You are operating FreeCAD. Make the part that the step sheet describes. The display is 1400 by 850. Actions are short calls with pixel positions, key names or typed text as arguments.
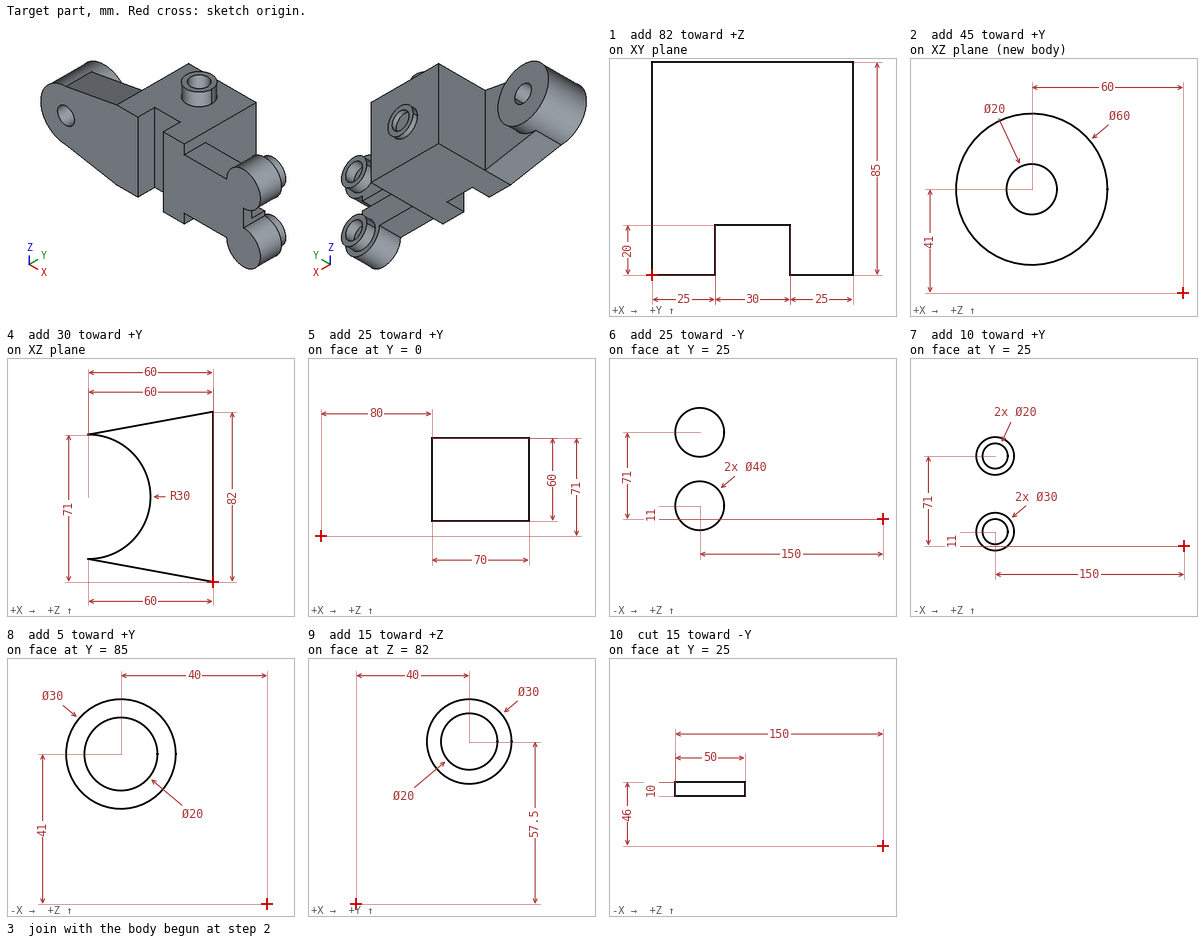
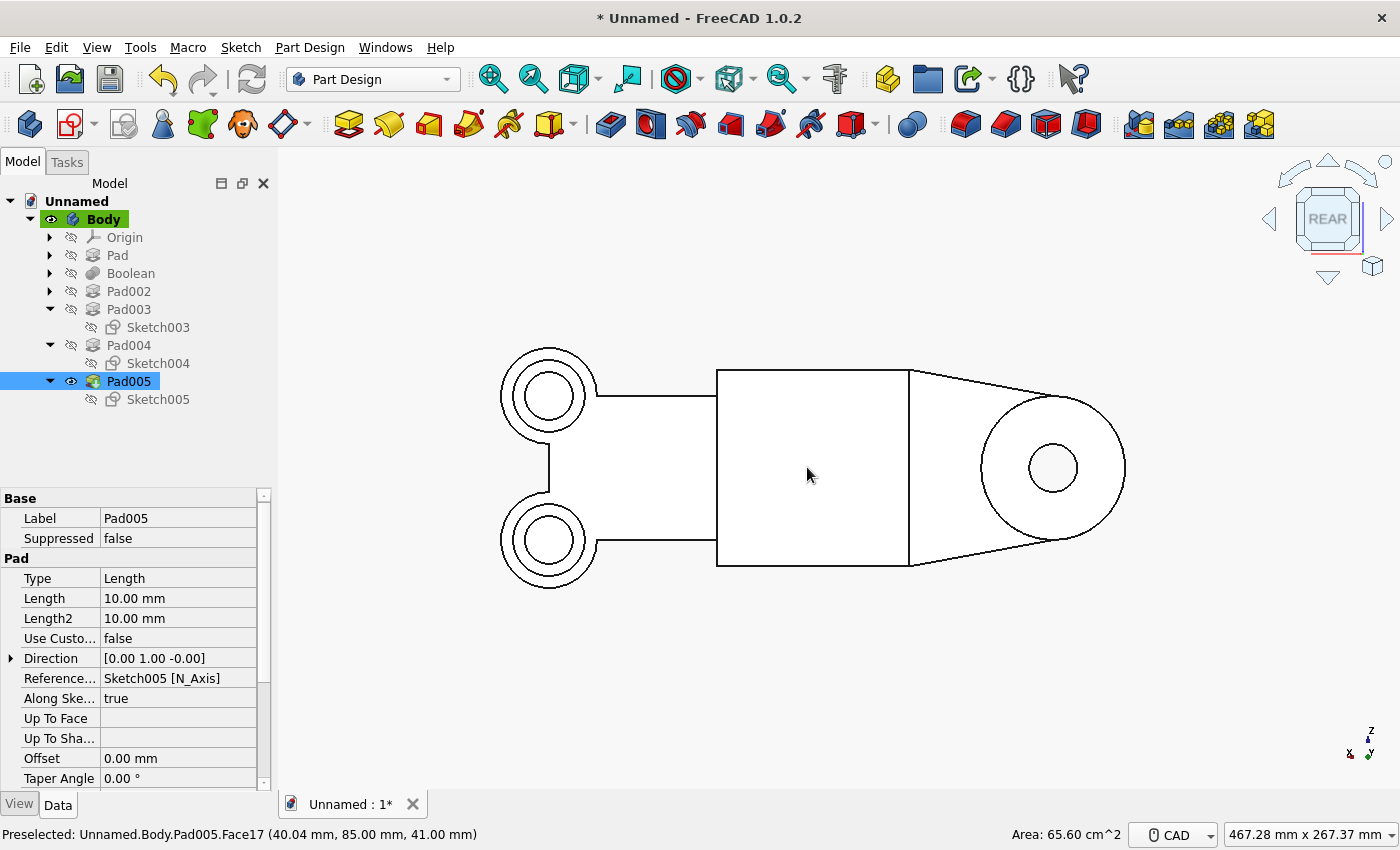
click(70, 124)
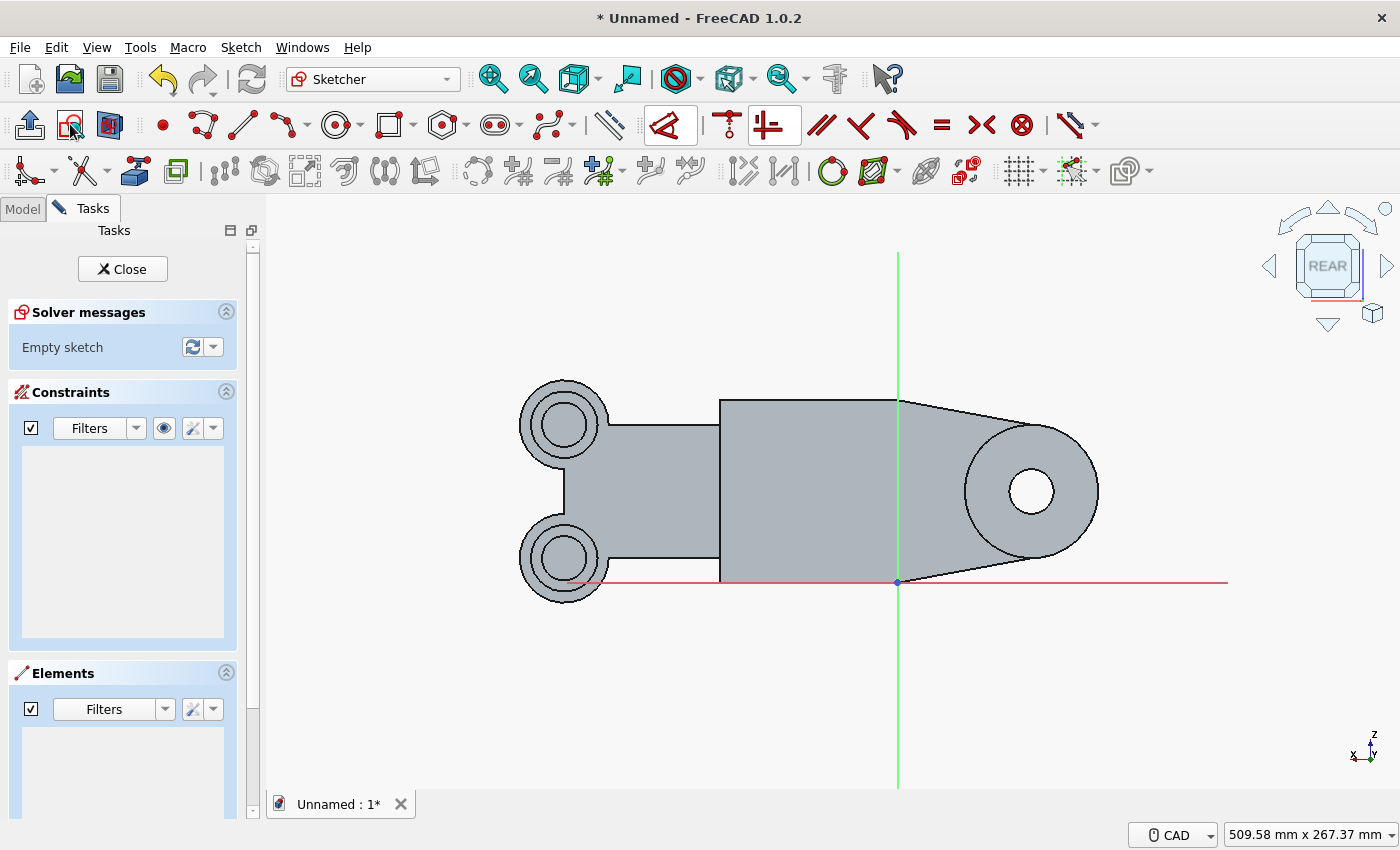
scroll(868, 533, up, 6)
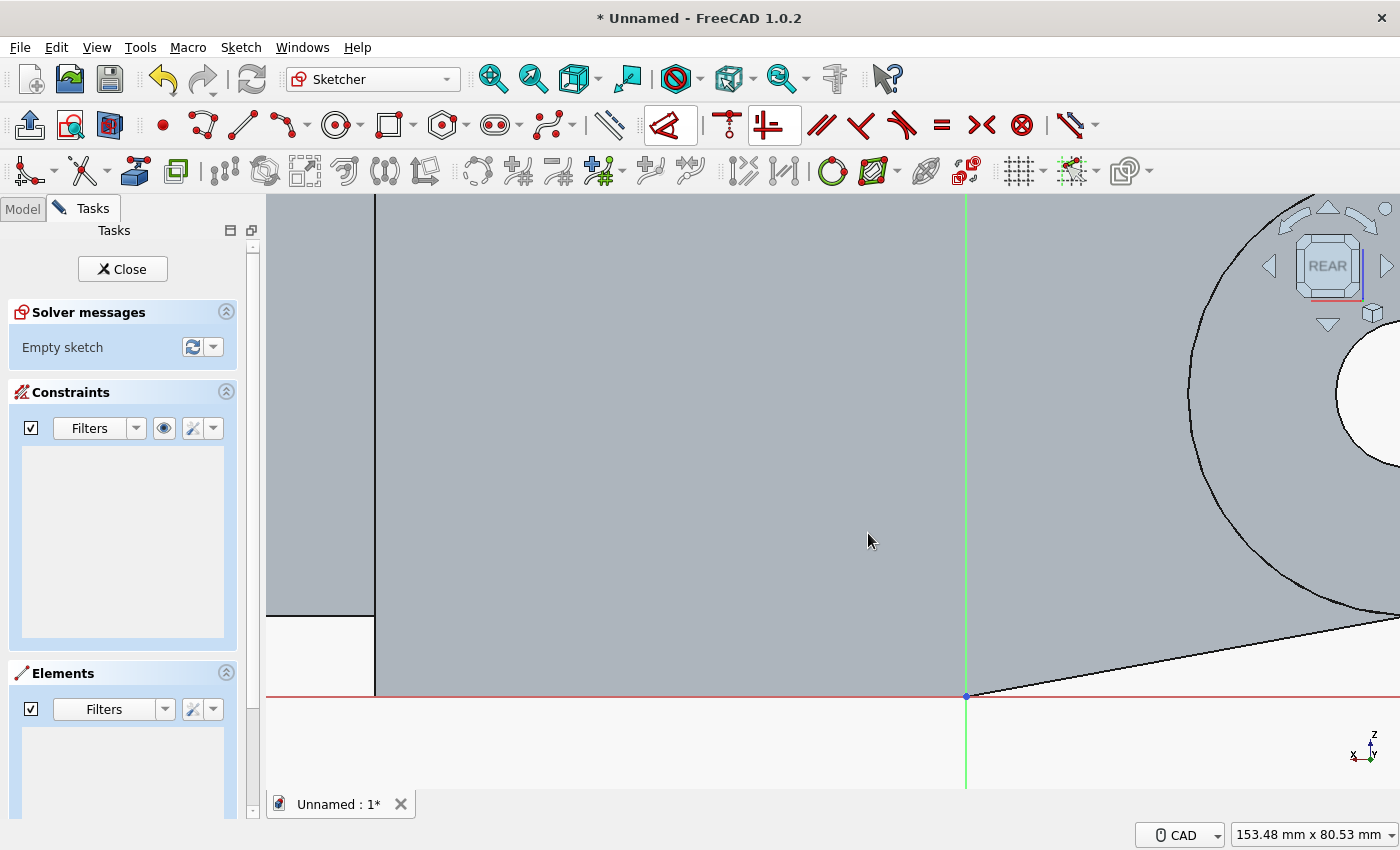
click(336, 126)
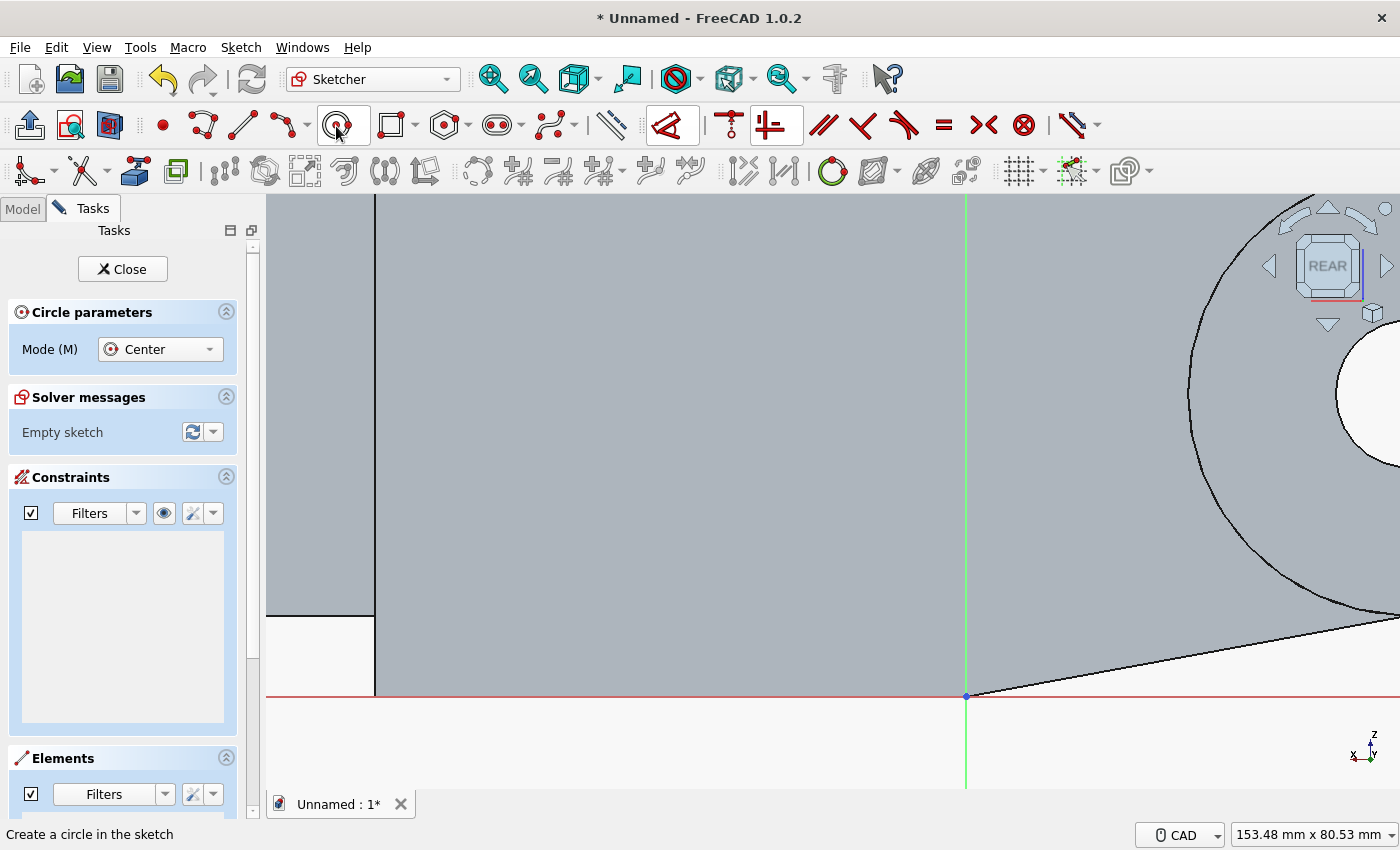
click(671, 394)
click(749, 316)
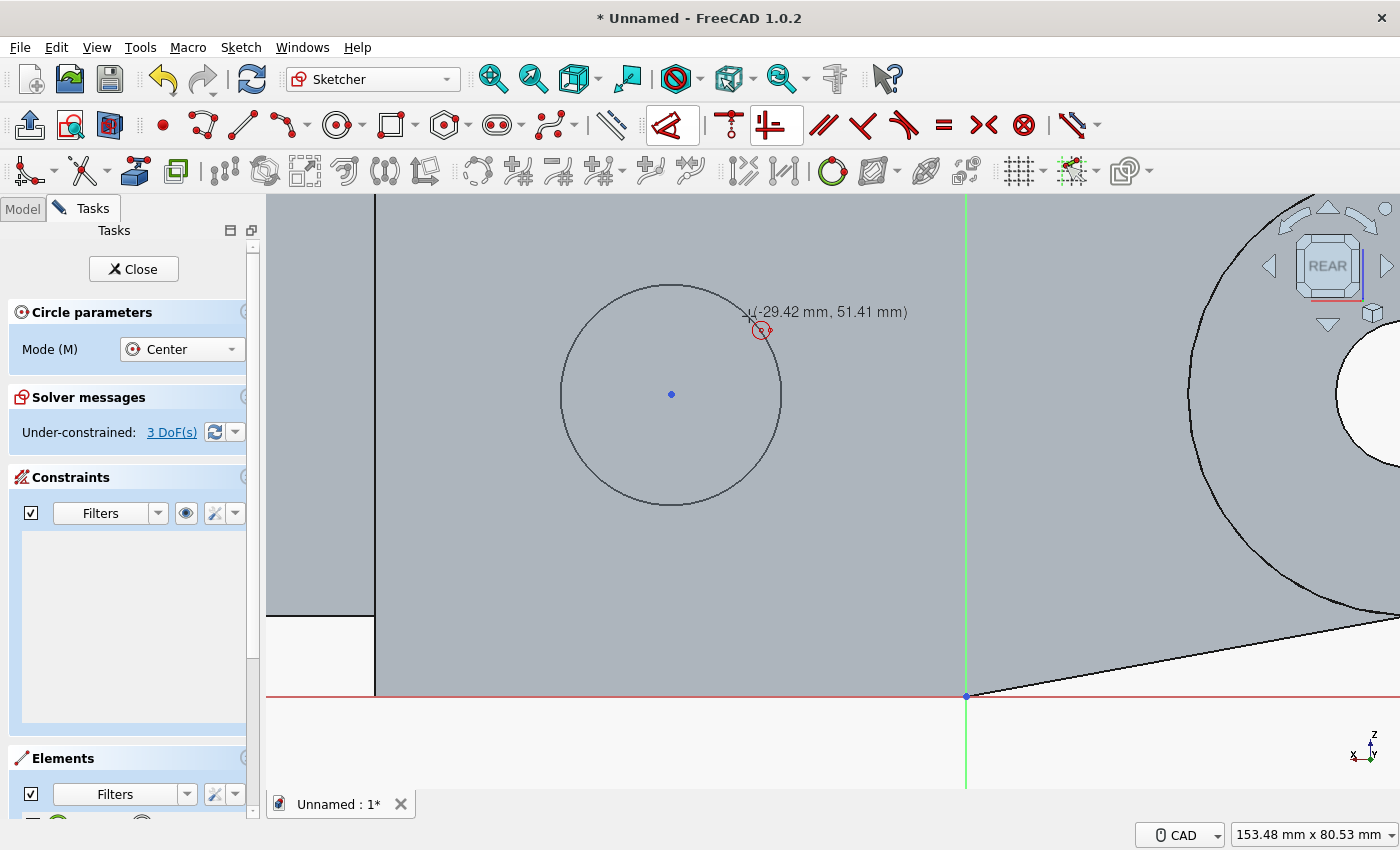
click(671, 395)
click(723, 342)
key(Escape)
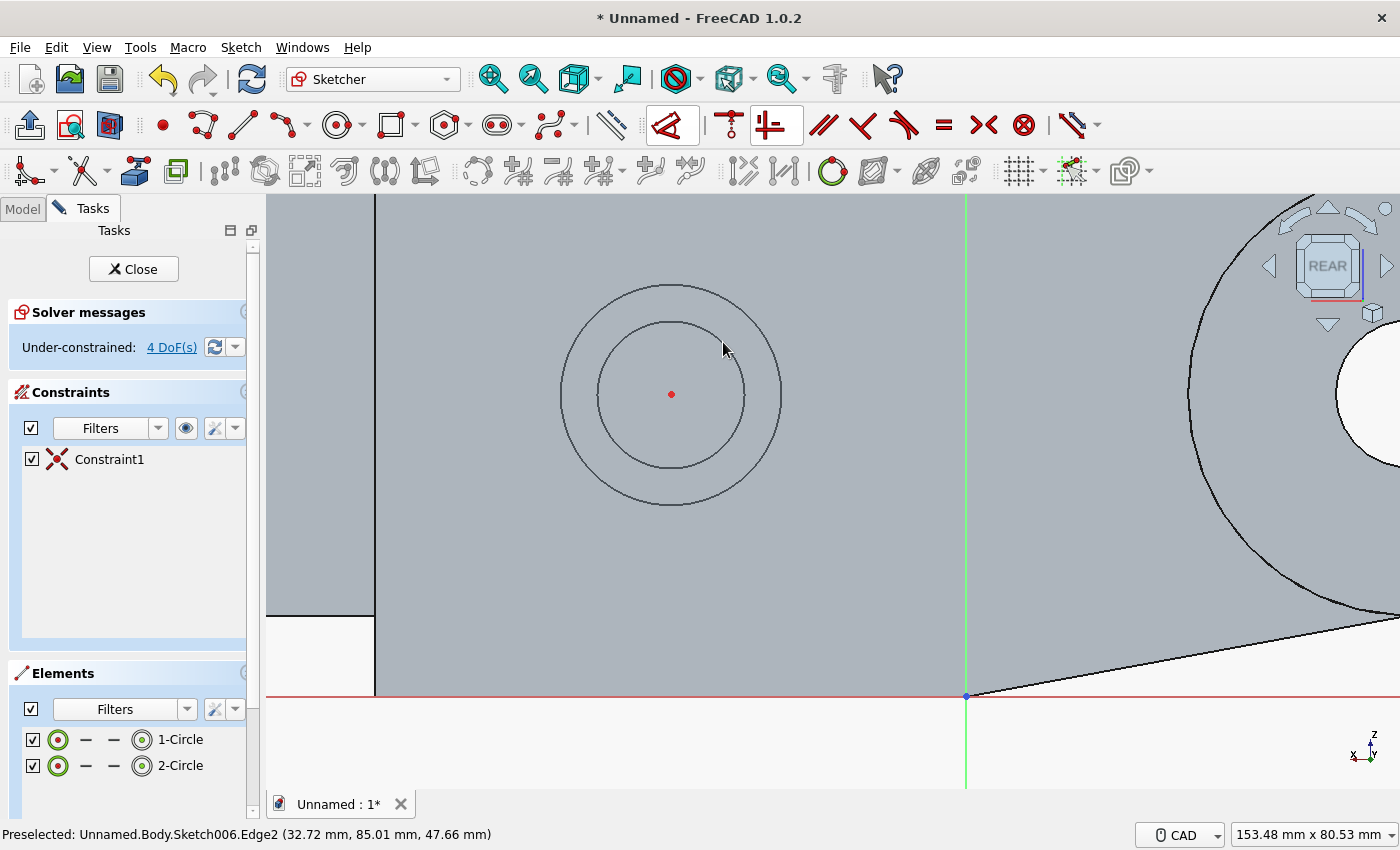
click(749, 317)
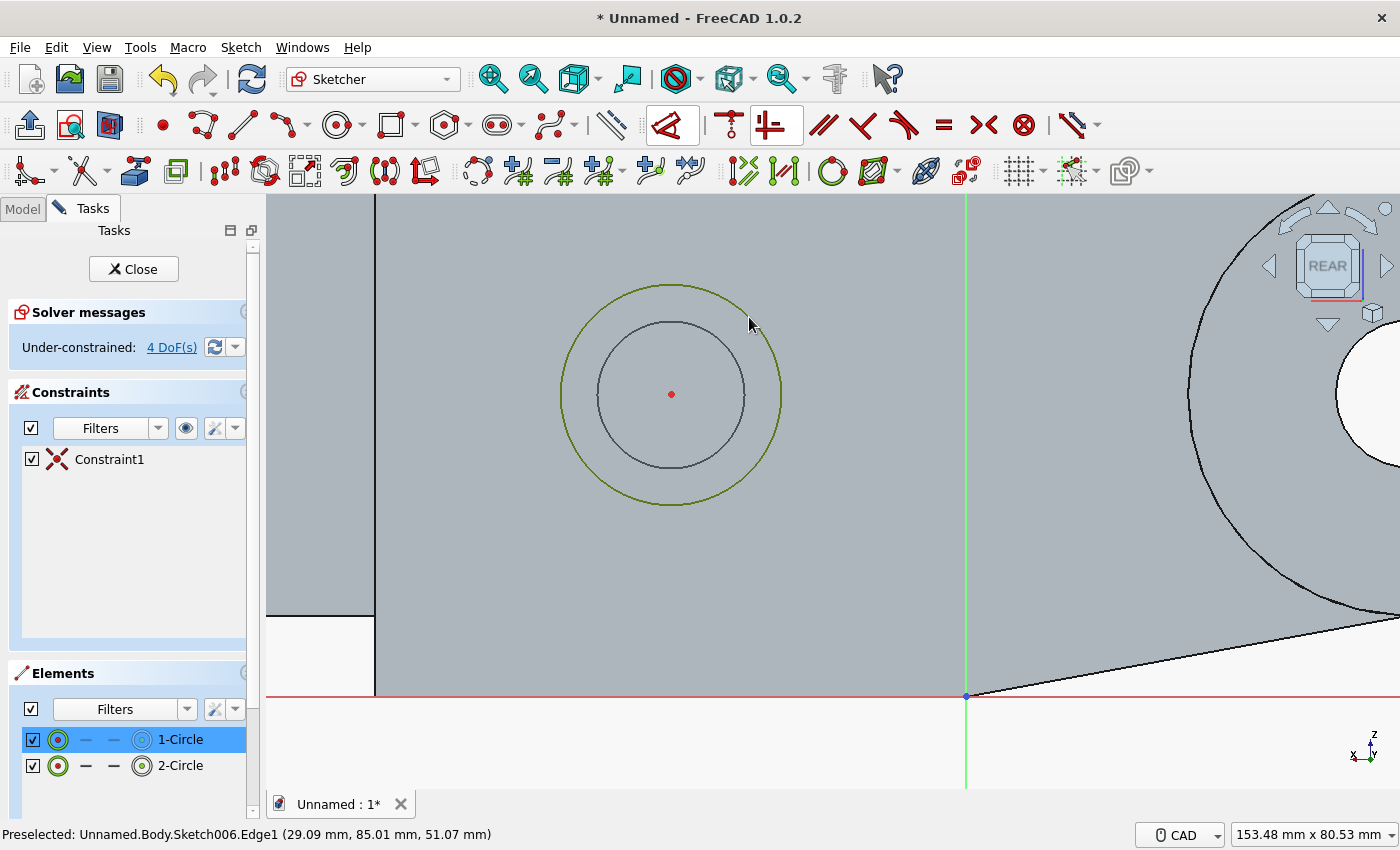
key(k)
key(o)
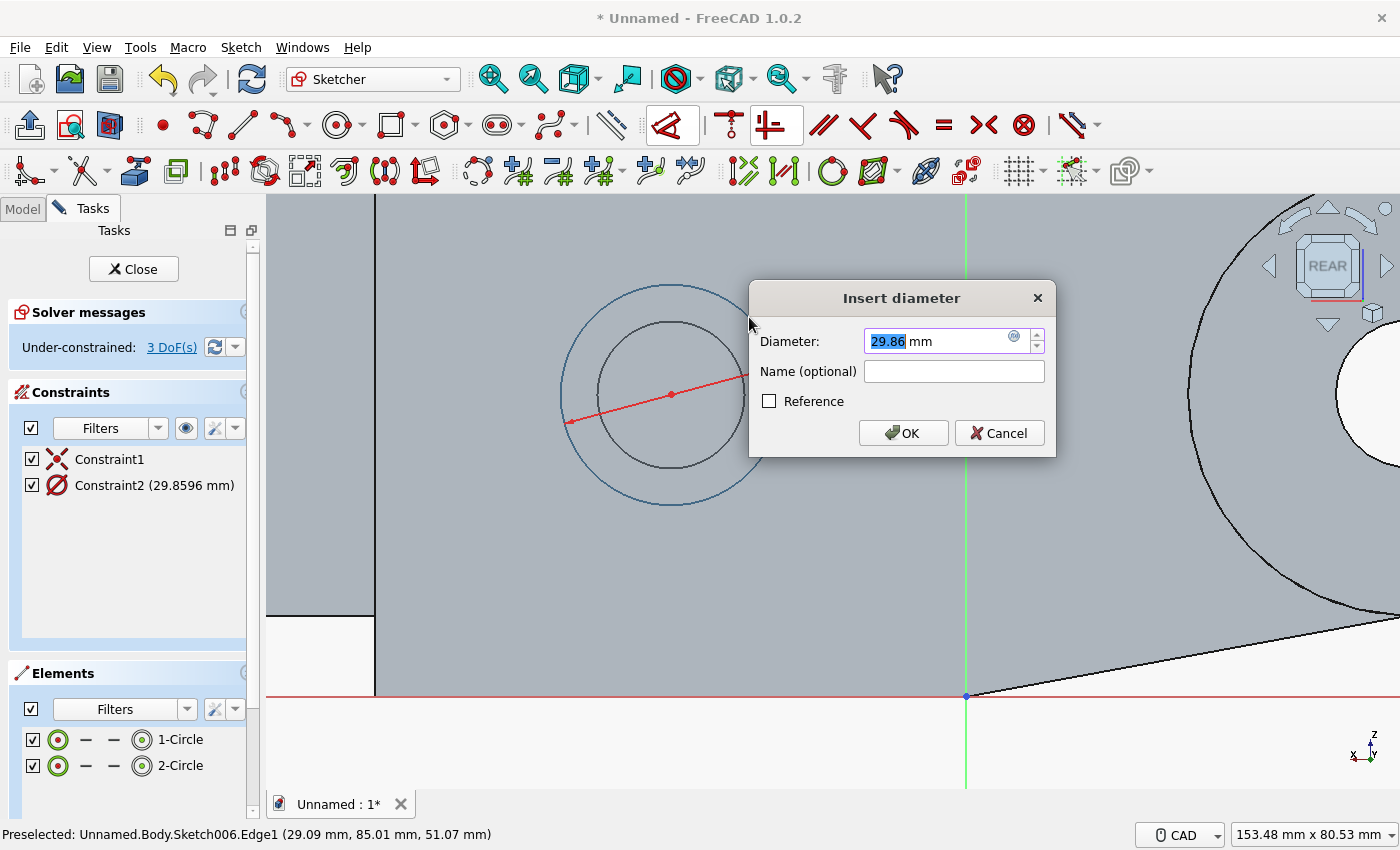
text(30)
key(Return)